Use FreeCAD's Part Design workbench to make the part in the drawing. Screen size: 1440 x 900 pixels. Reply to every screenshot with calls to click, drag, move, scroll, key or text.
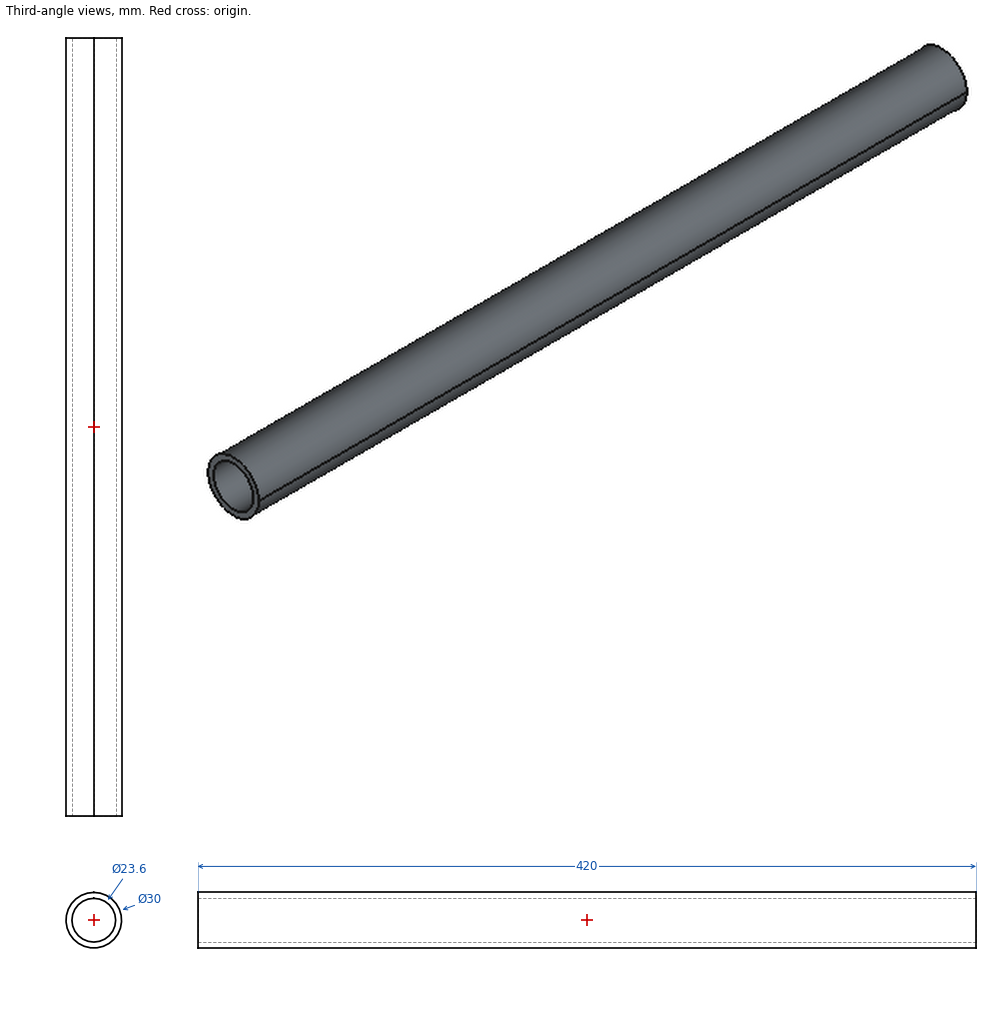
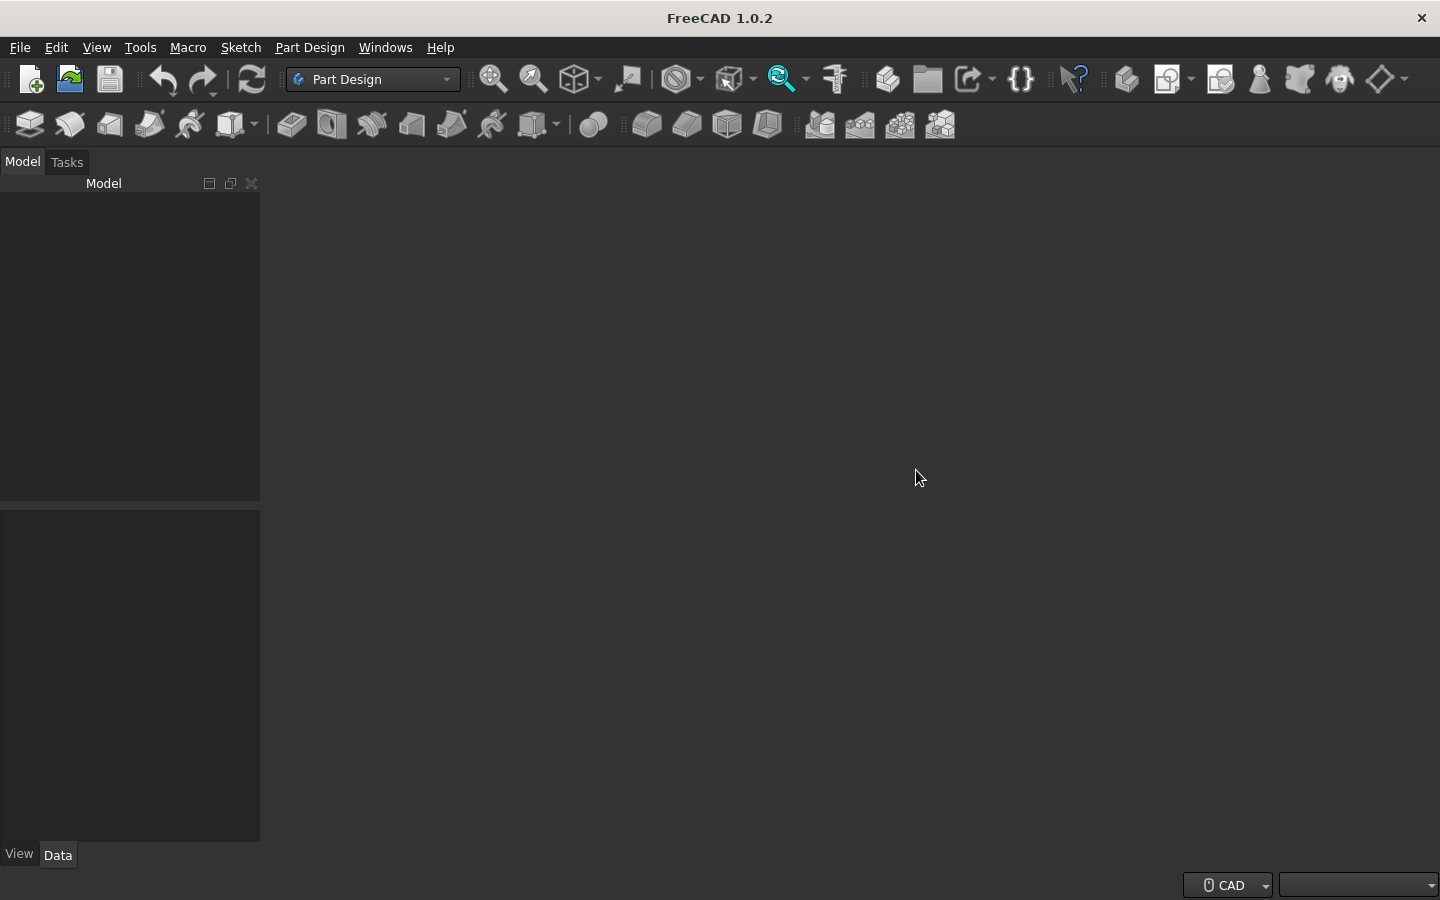
click(30, 80)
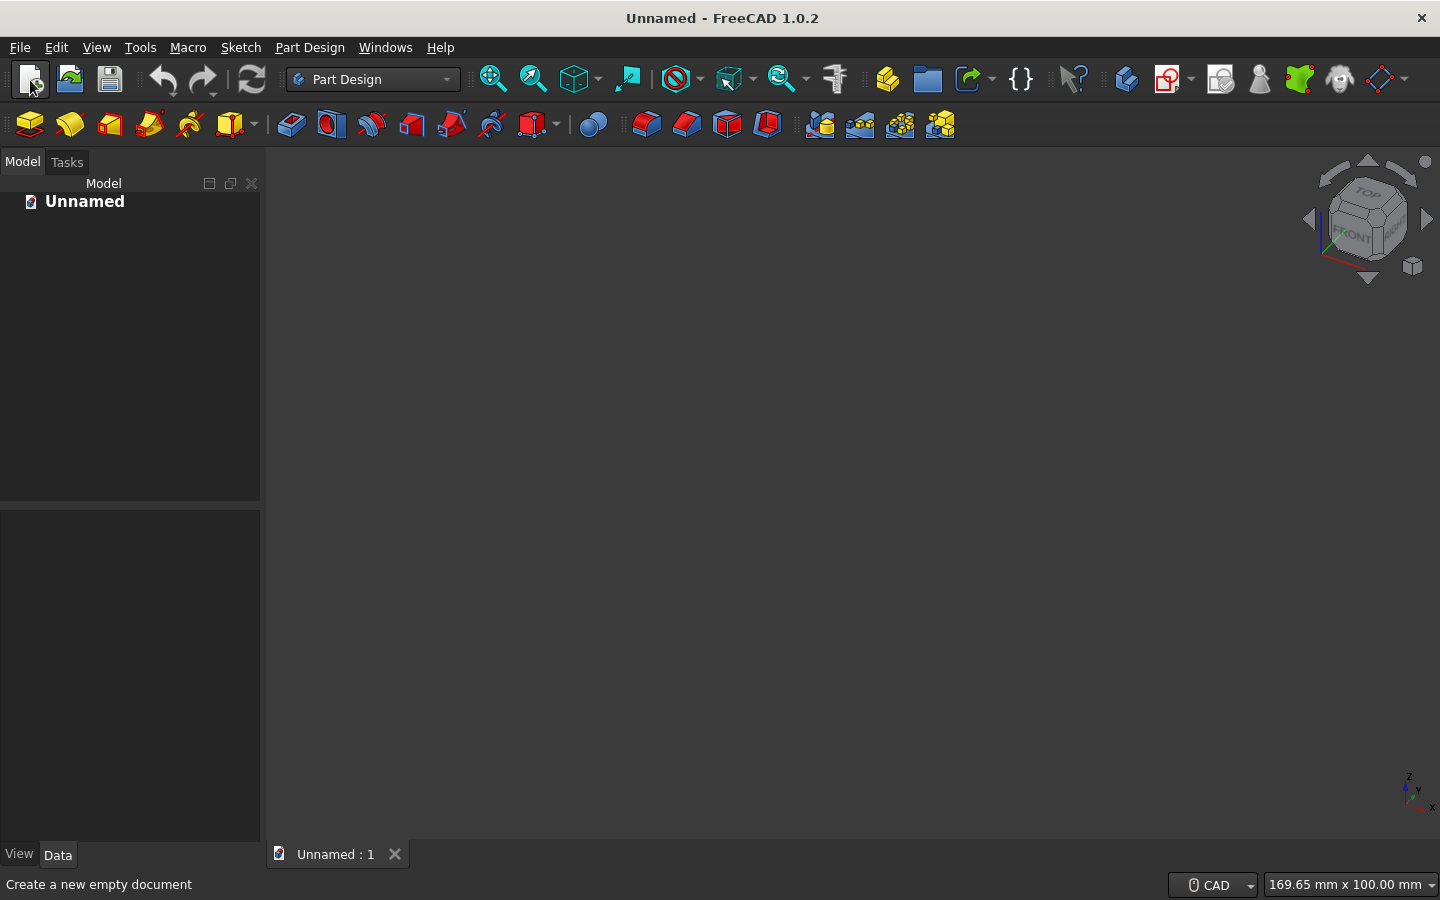
click(1168, 80)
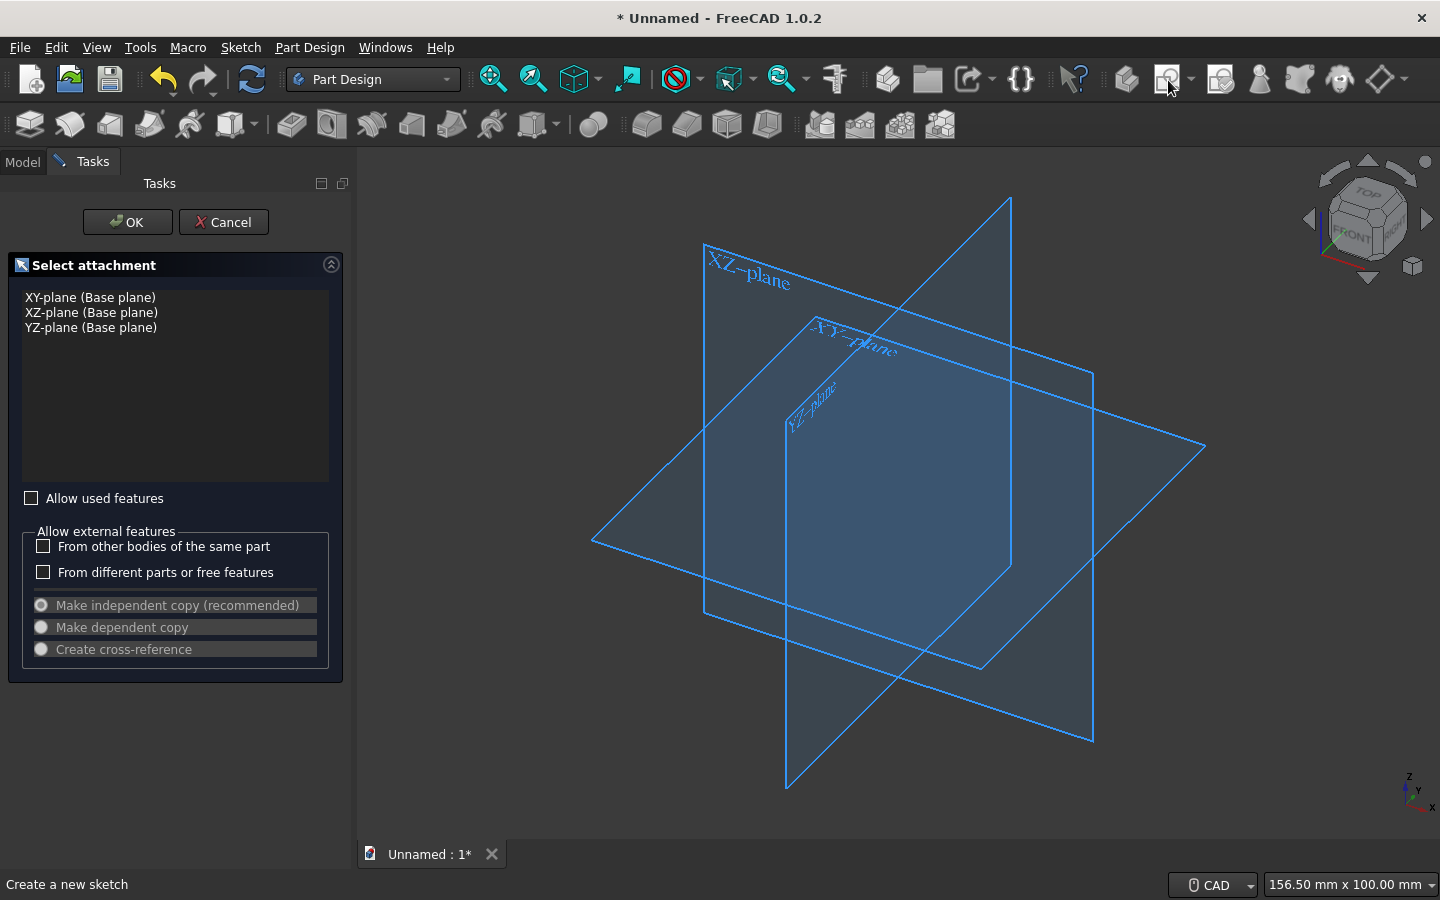
click(82, 312)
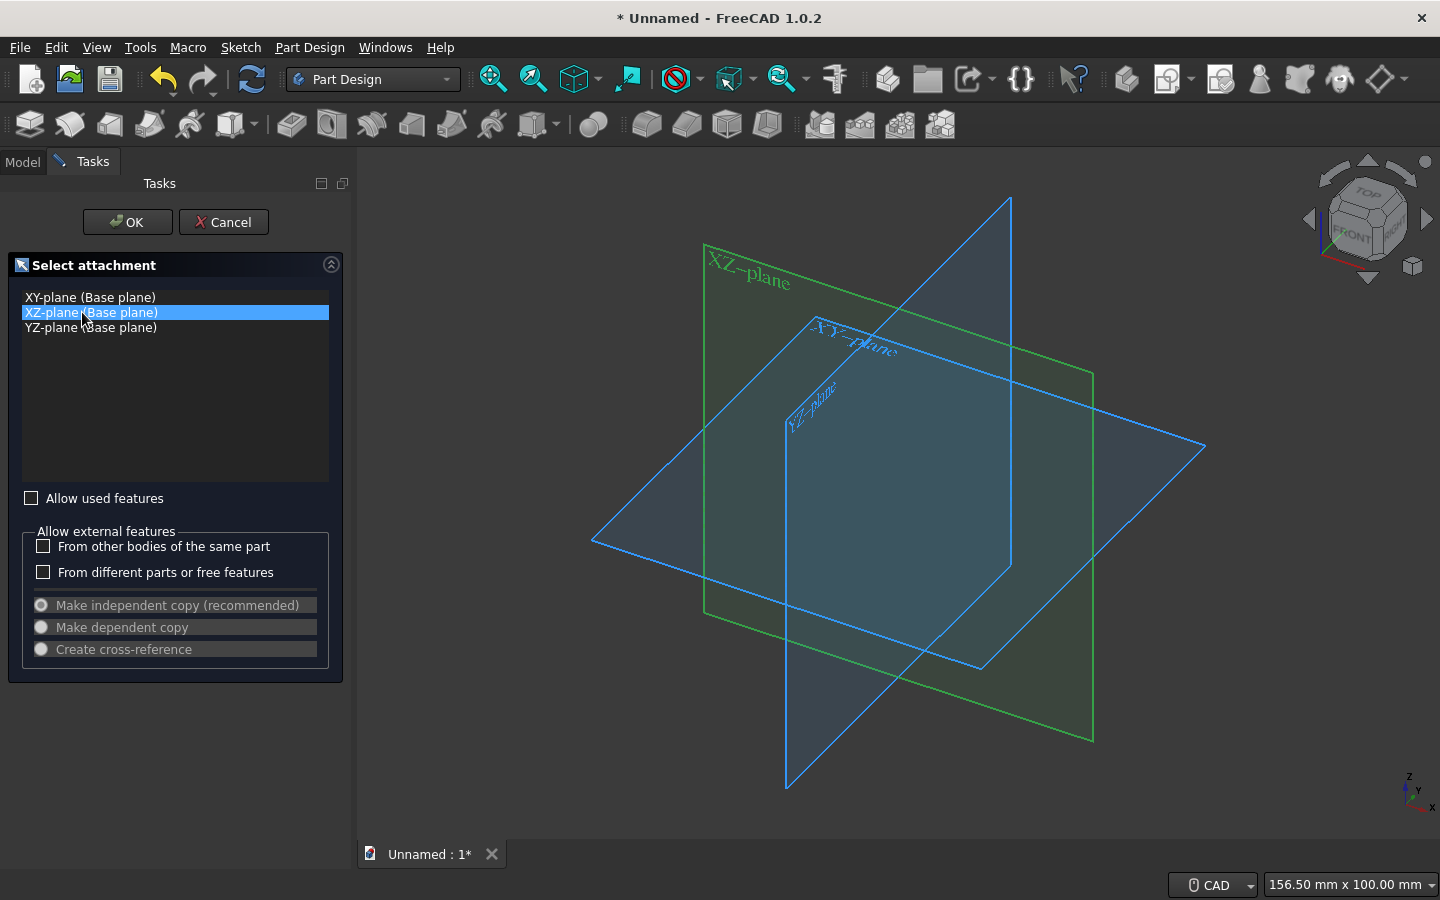
click(128, 222)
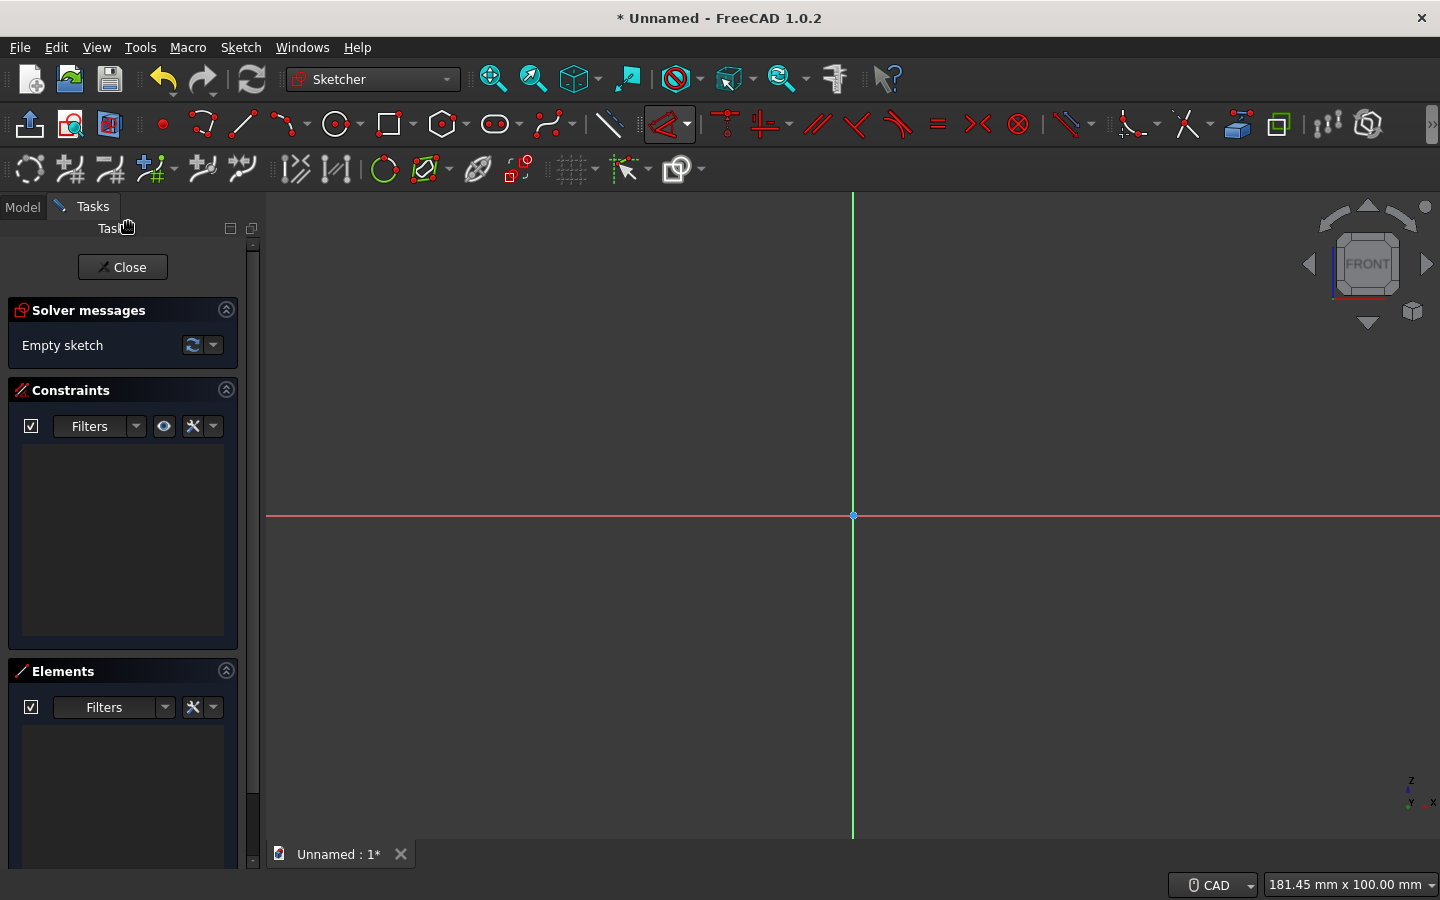
scroll(909, 516, up, 4)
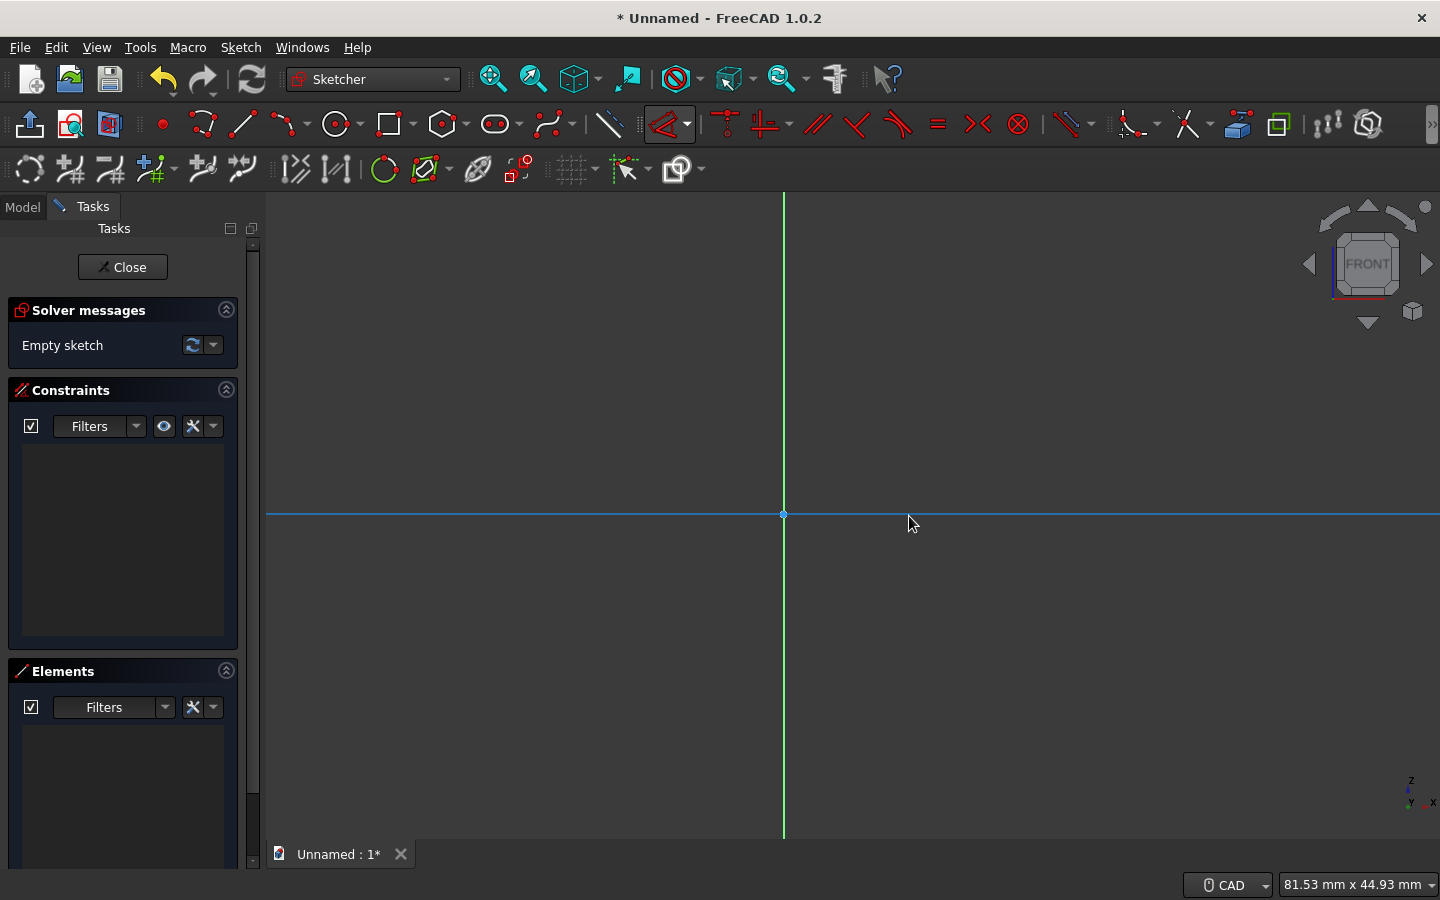
click(336, 124)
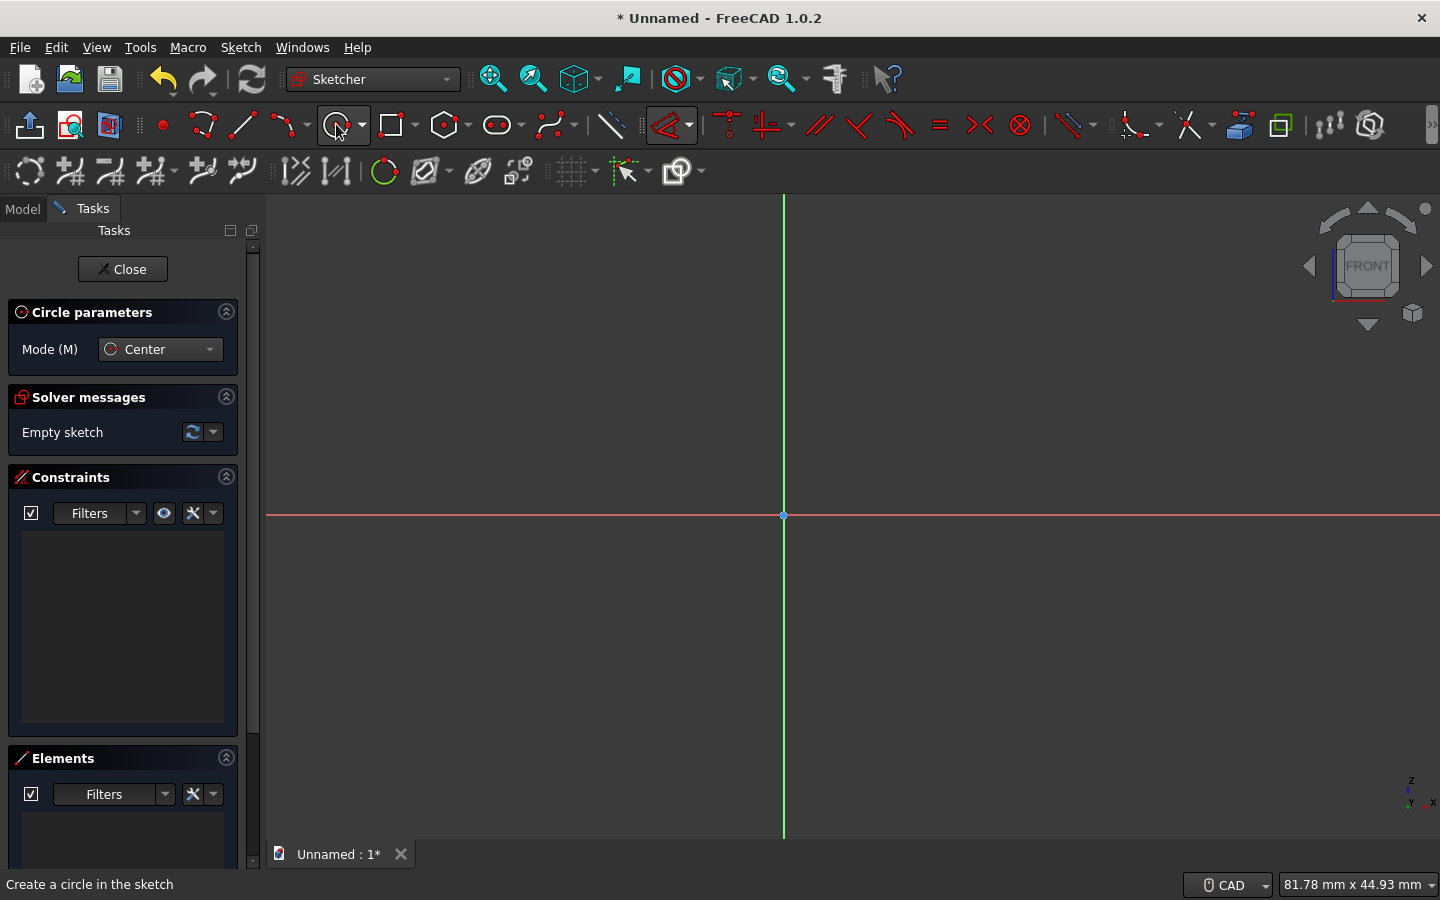
click(784, 515)
click(936, 363)